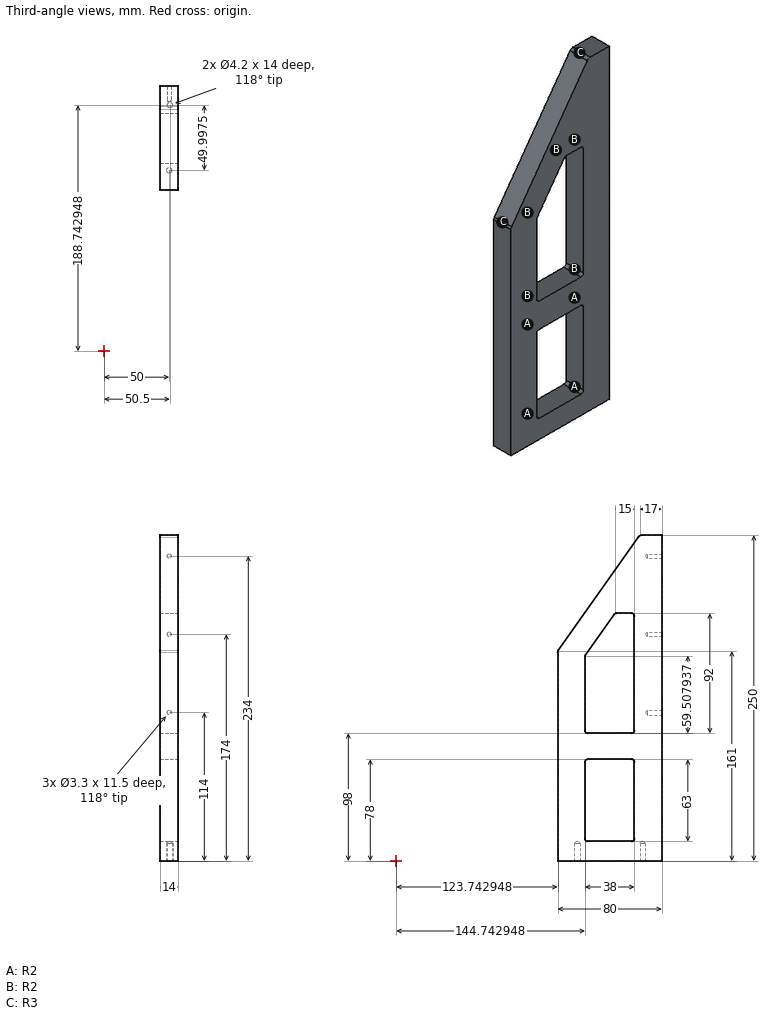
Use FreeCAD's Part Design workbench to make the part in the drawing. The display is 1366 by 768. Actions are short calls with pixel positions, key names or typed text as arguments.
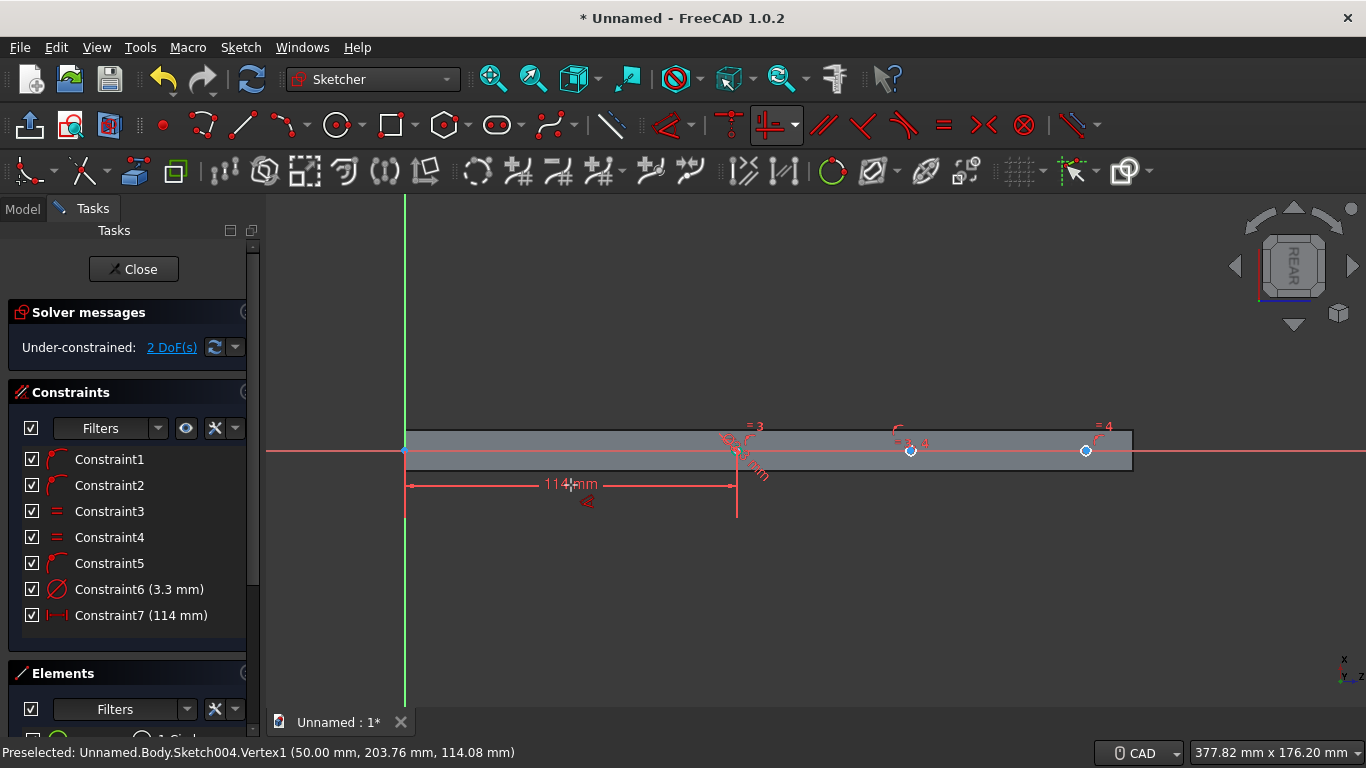
click(911, 451)
click(658, 485)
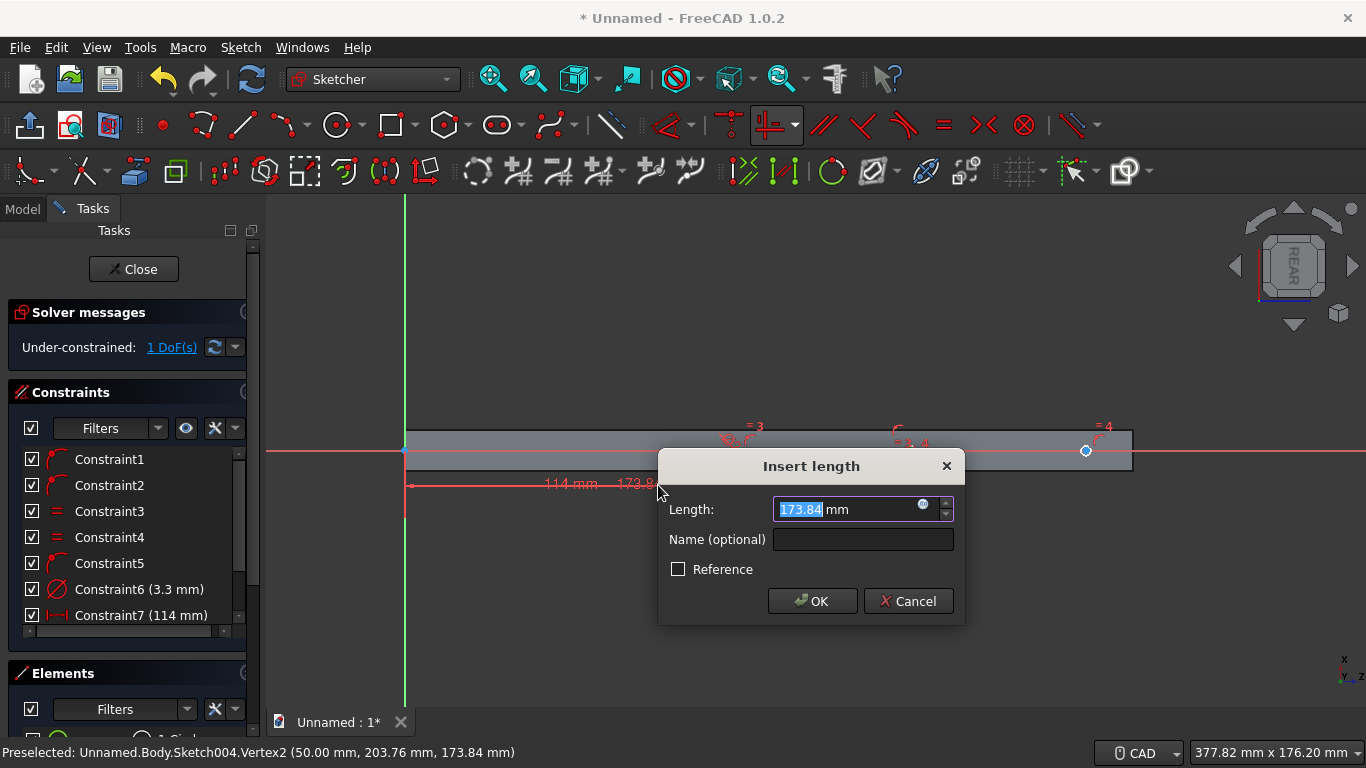
text(174)
key(Return)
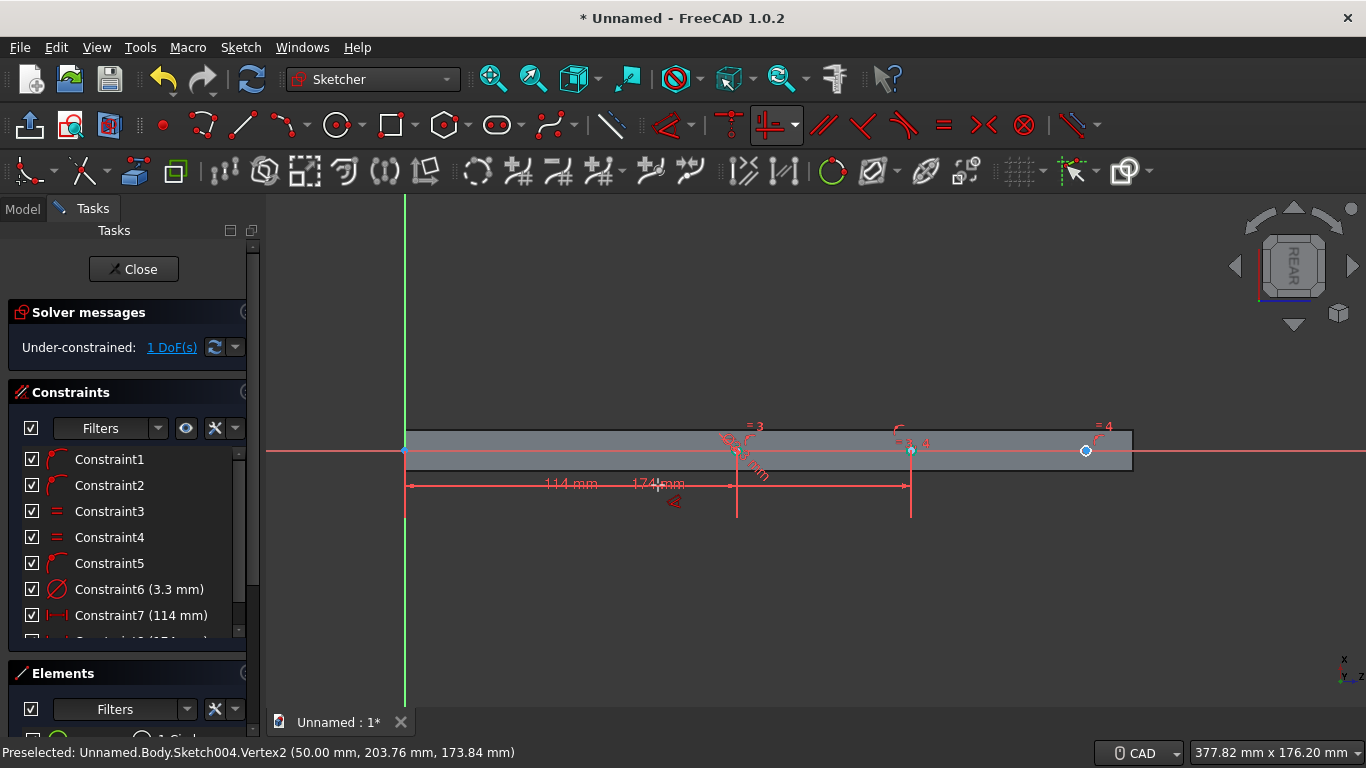
click(1086, 451)
click(745, 485)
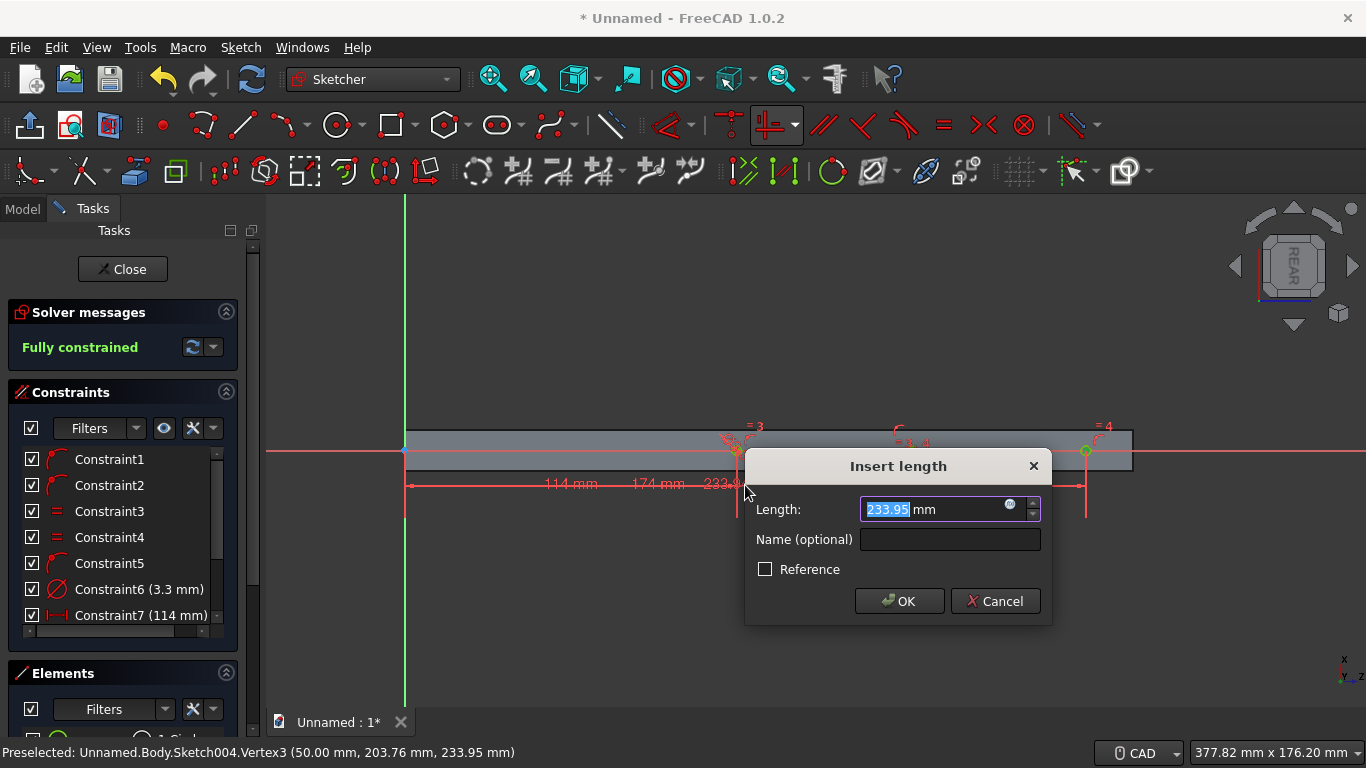
text(234)
key(Return)
key(Escape)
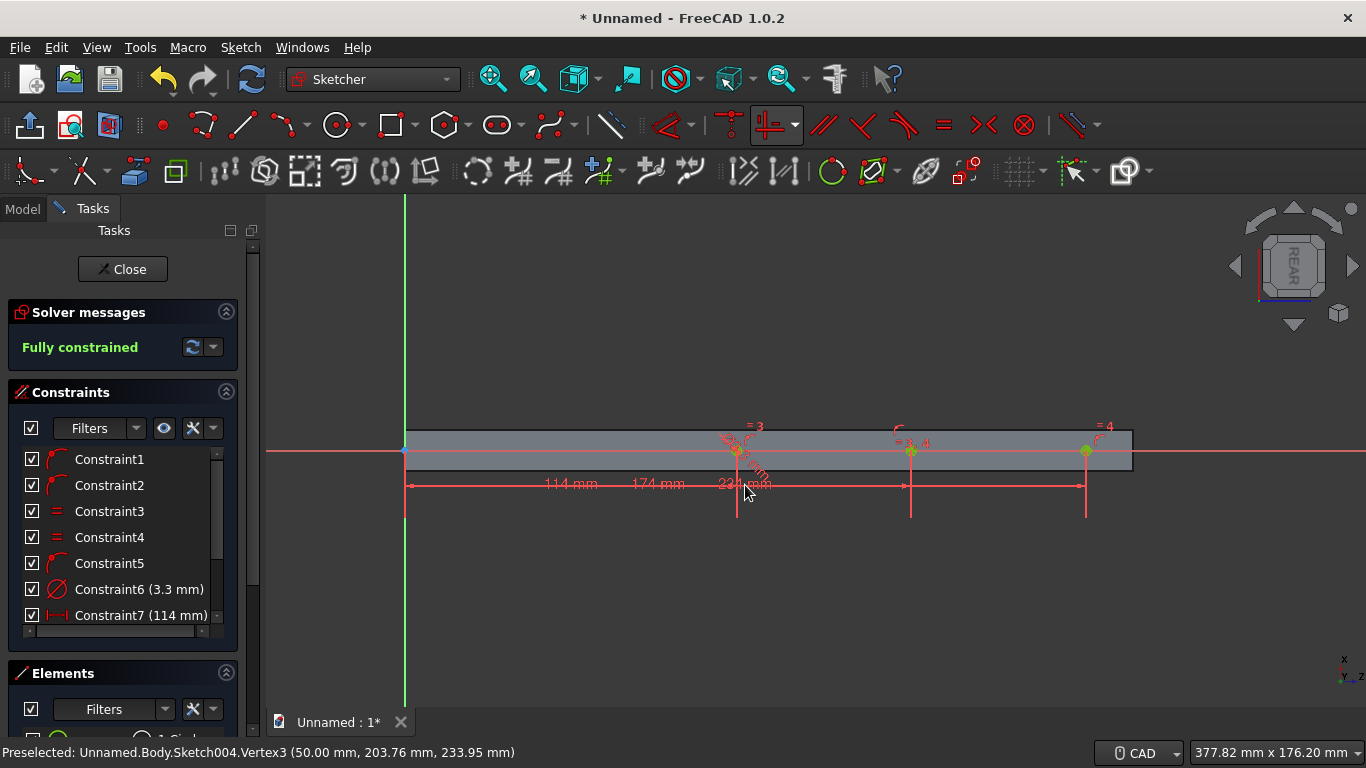
click(123, 269)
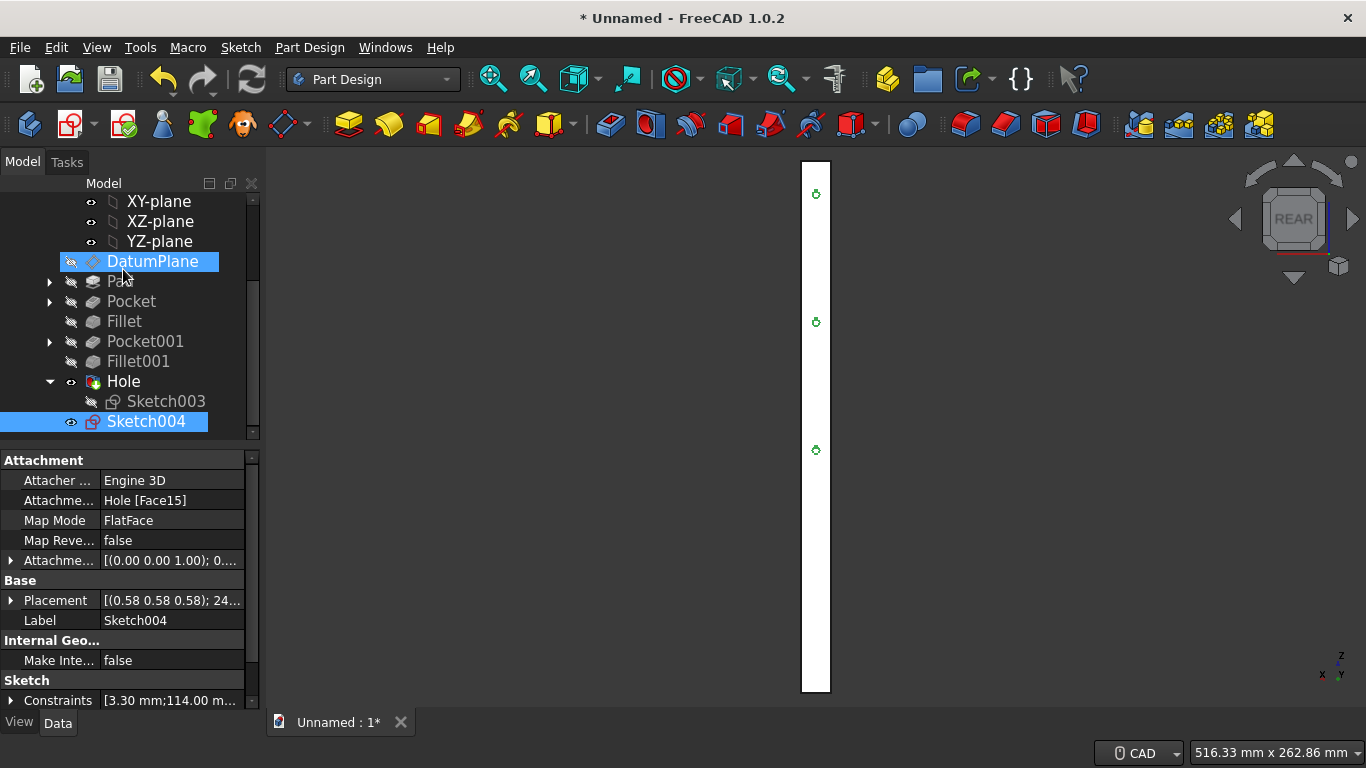
click(652, 124)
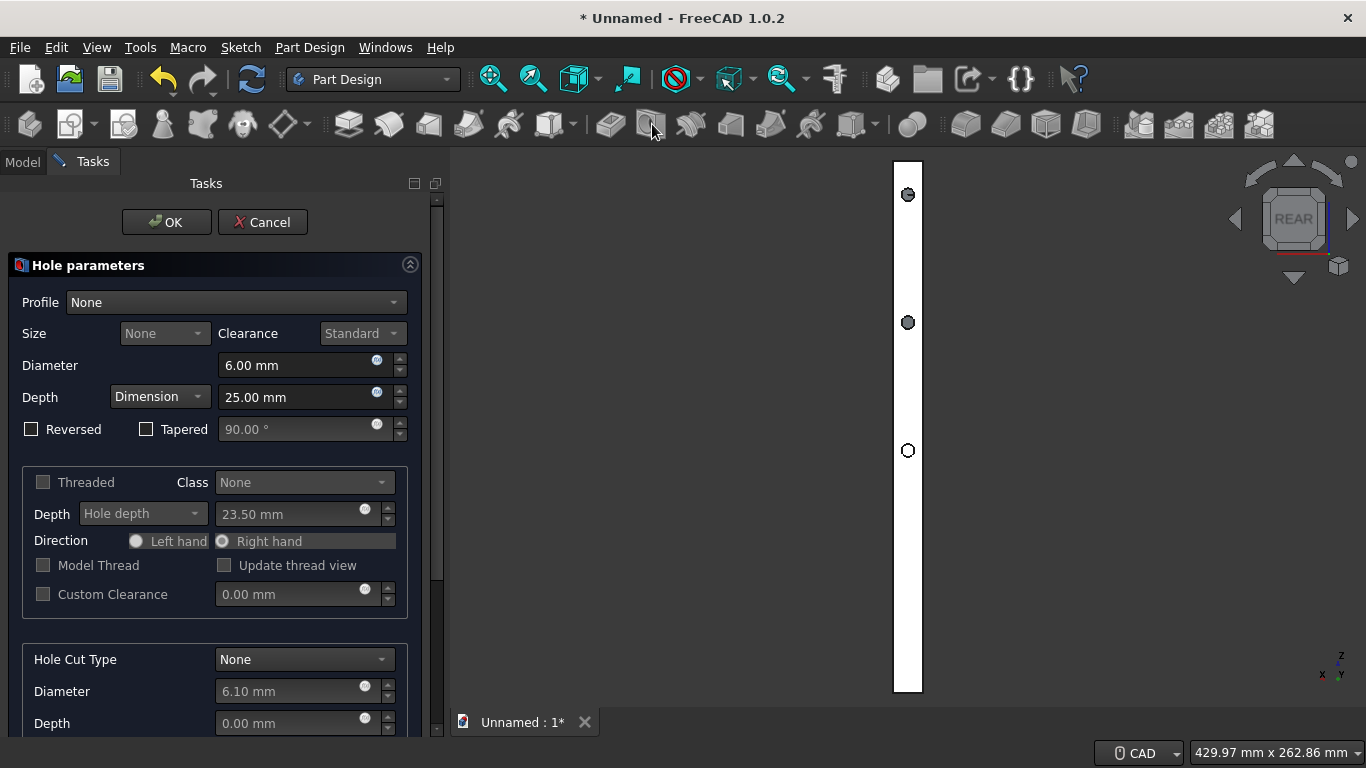
triple_click(305, 365)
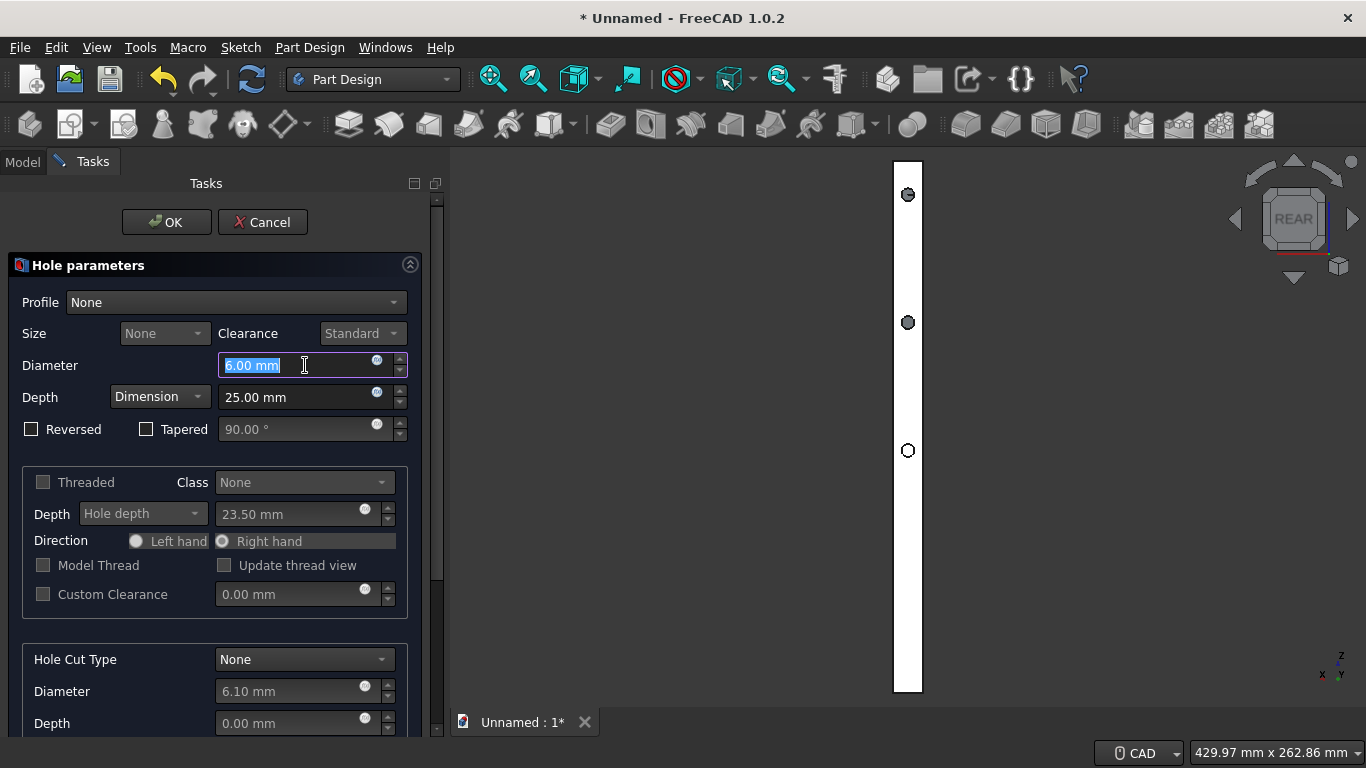
text(3.3)
key(Tab)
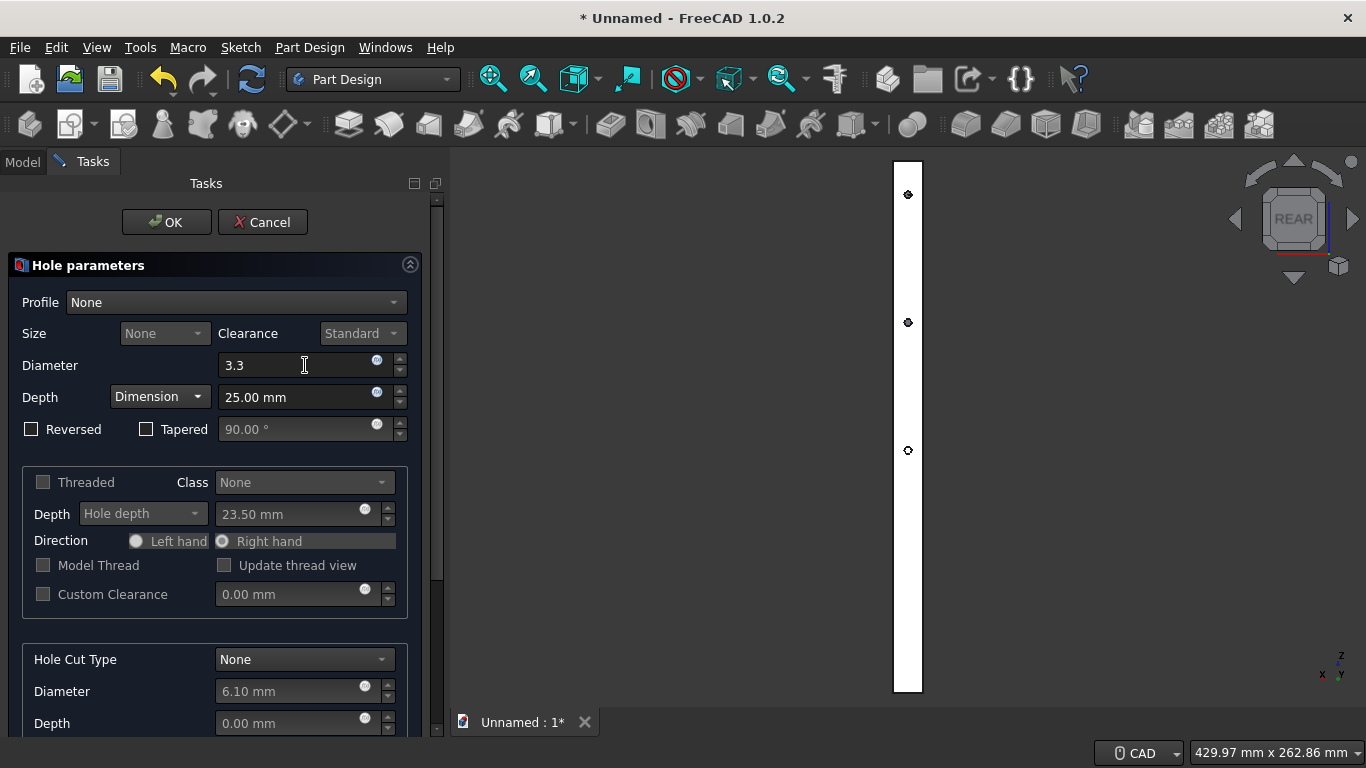
triple_click(305, 397)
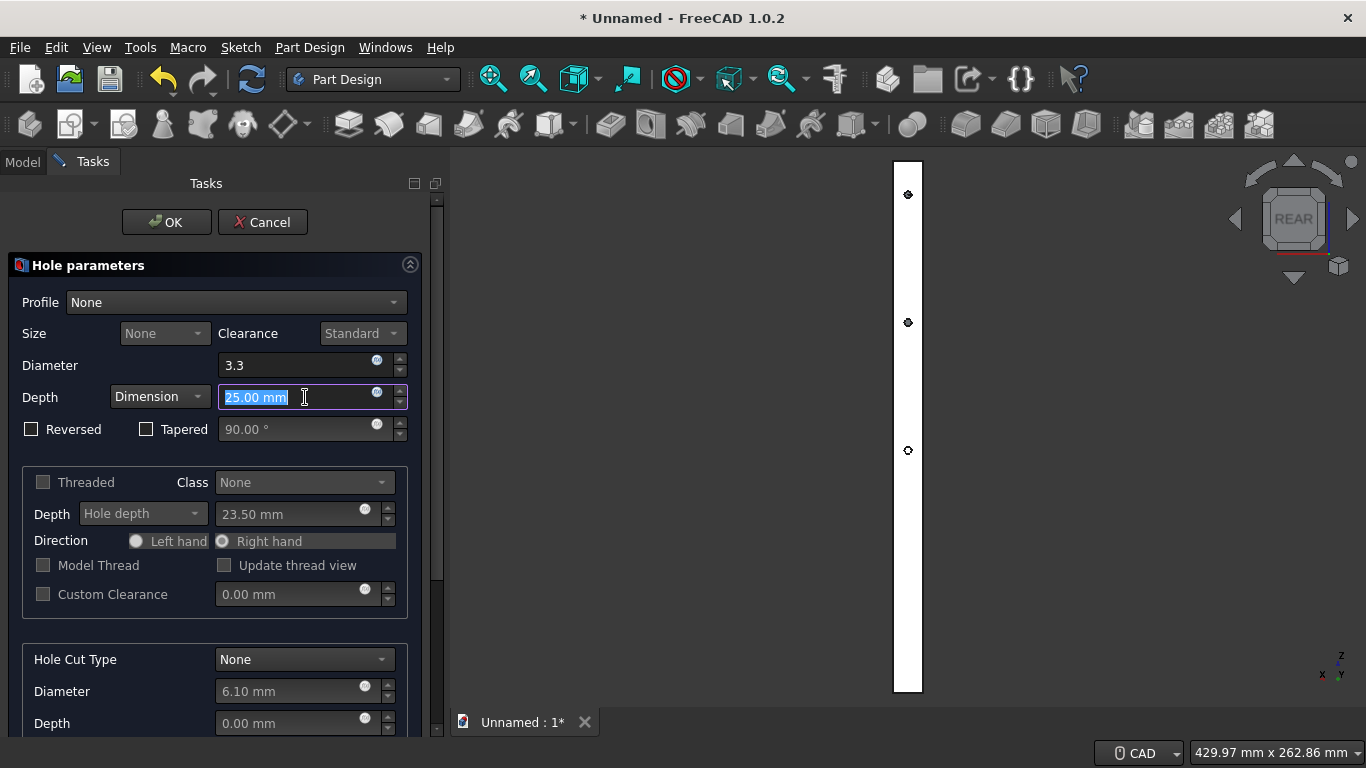
text(11.5)
key(Tab)